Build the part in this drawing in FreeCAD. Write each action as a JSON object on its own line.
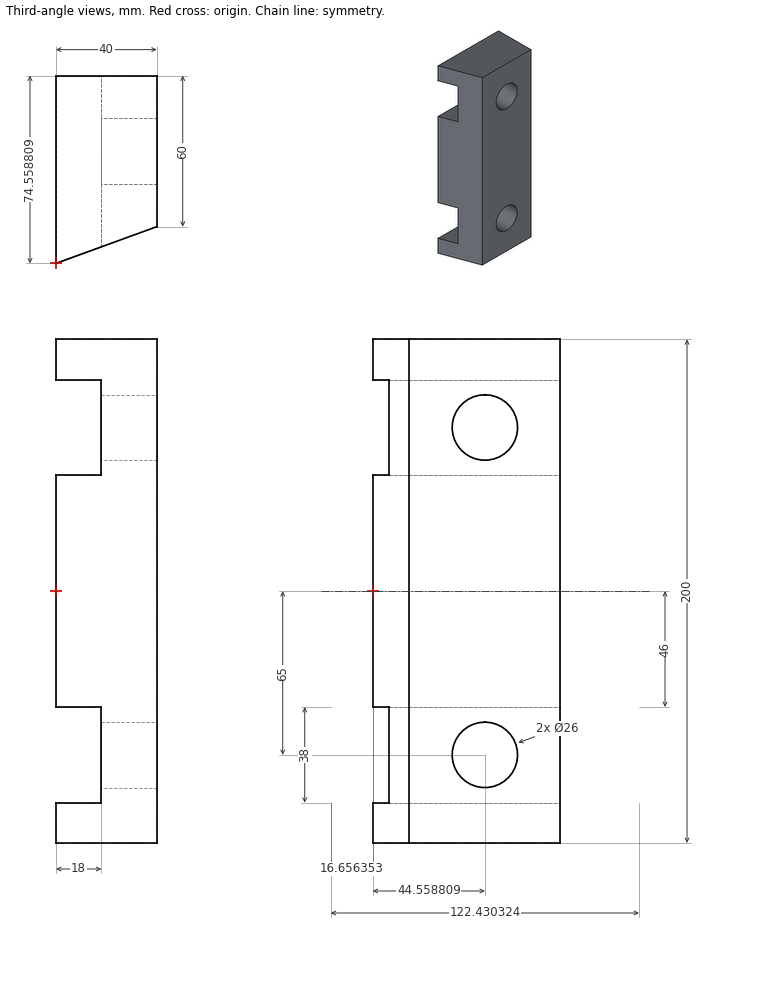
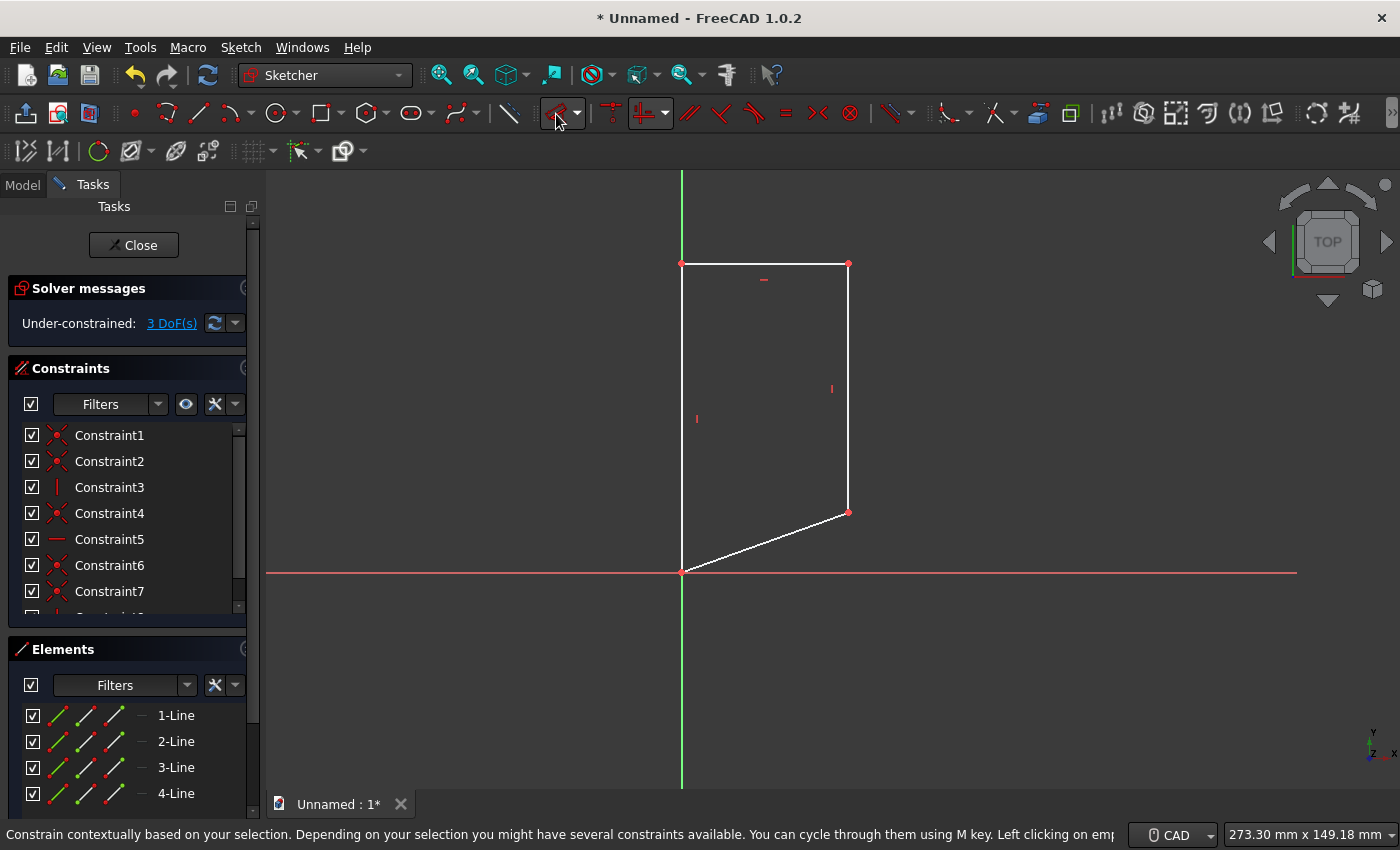
{"action": "left_click", "coordinate": [848, 438]}
{"action": "left_click", "coordinate": [882, 389]}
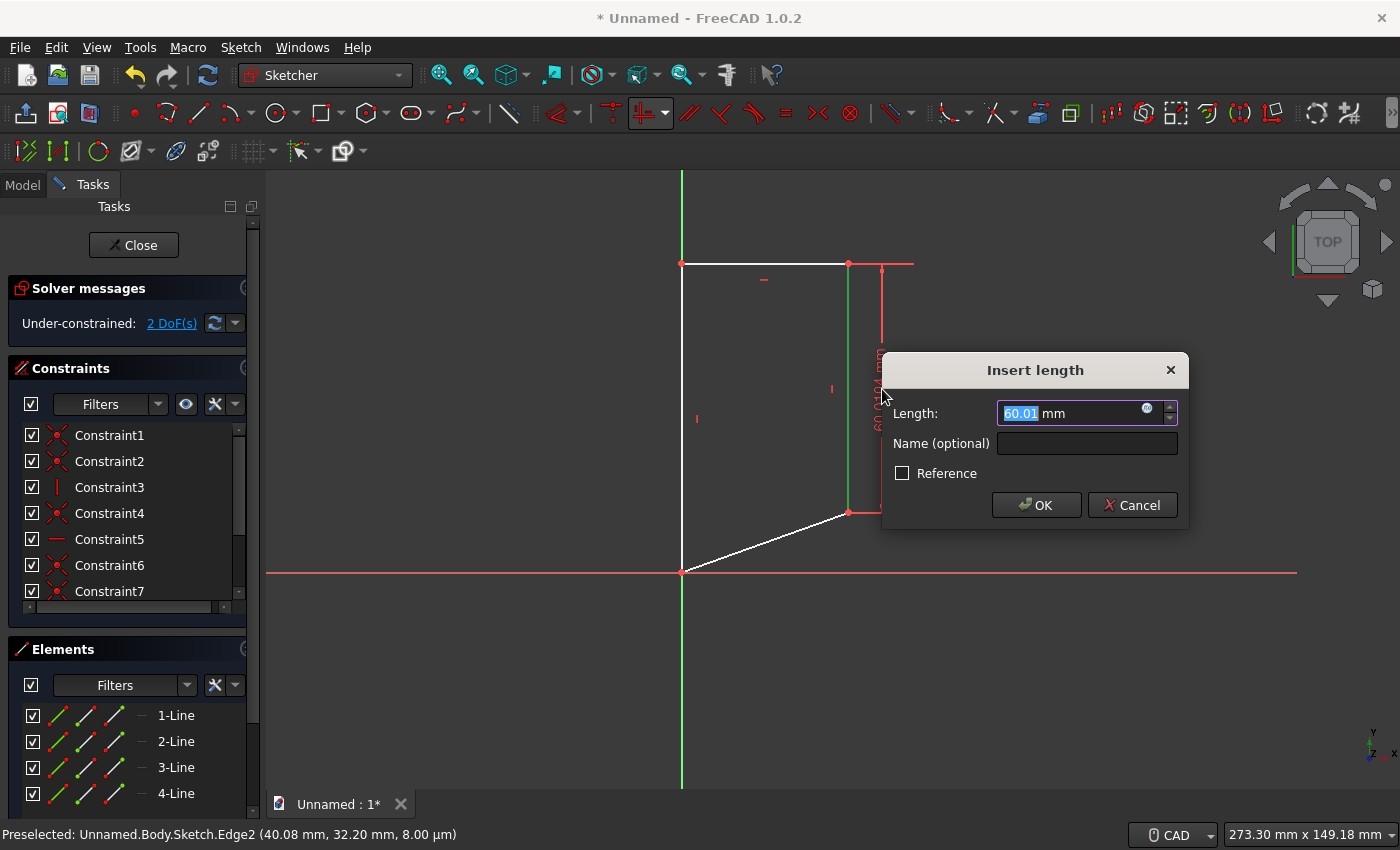
{"action": "type", "text": "60"}
{"action": "key", "text": "Return"}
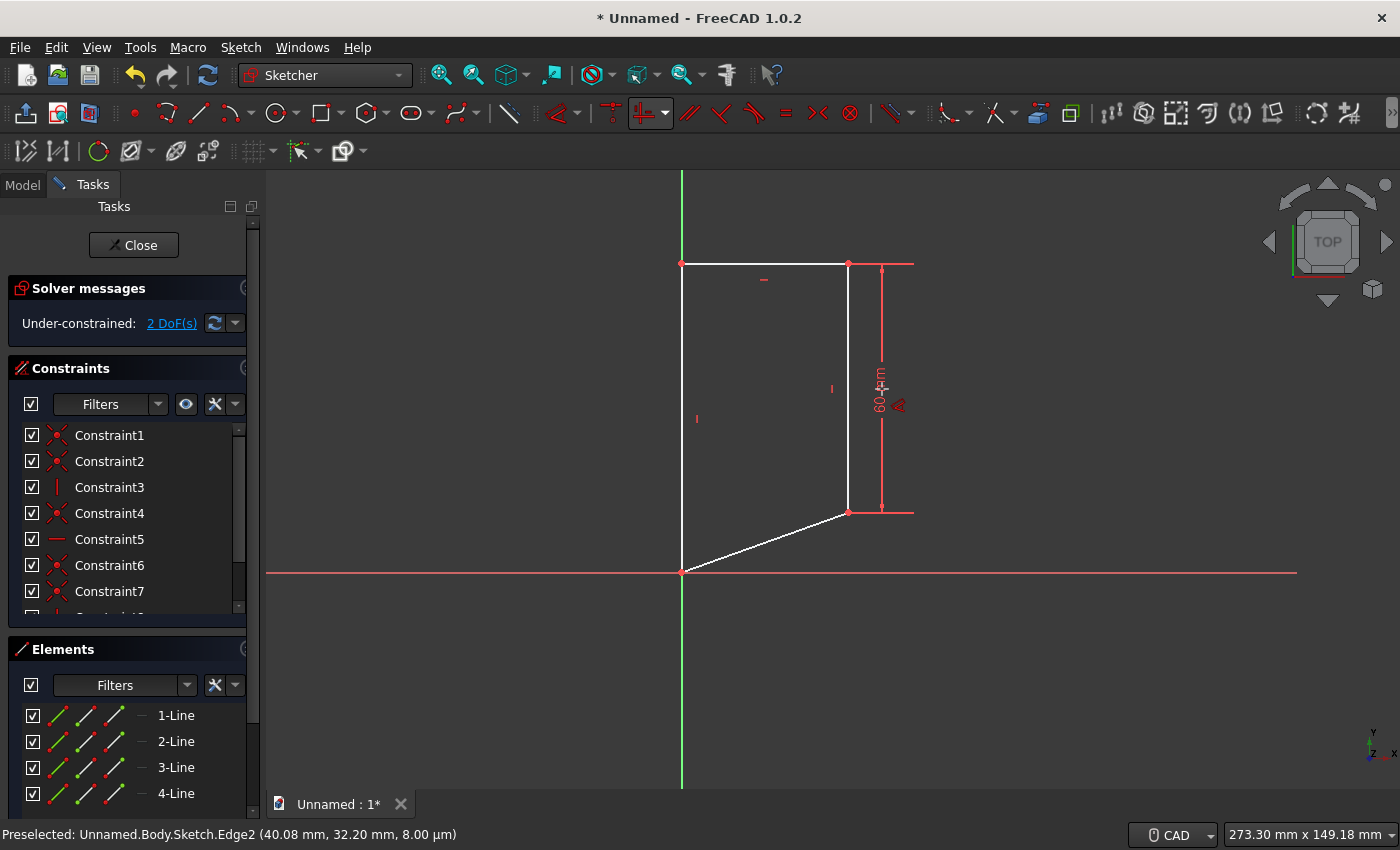
{"action": "left_click", "coordinate": [798, 264]}
{"action": "left_click", "coordinate": [765, 230]}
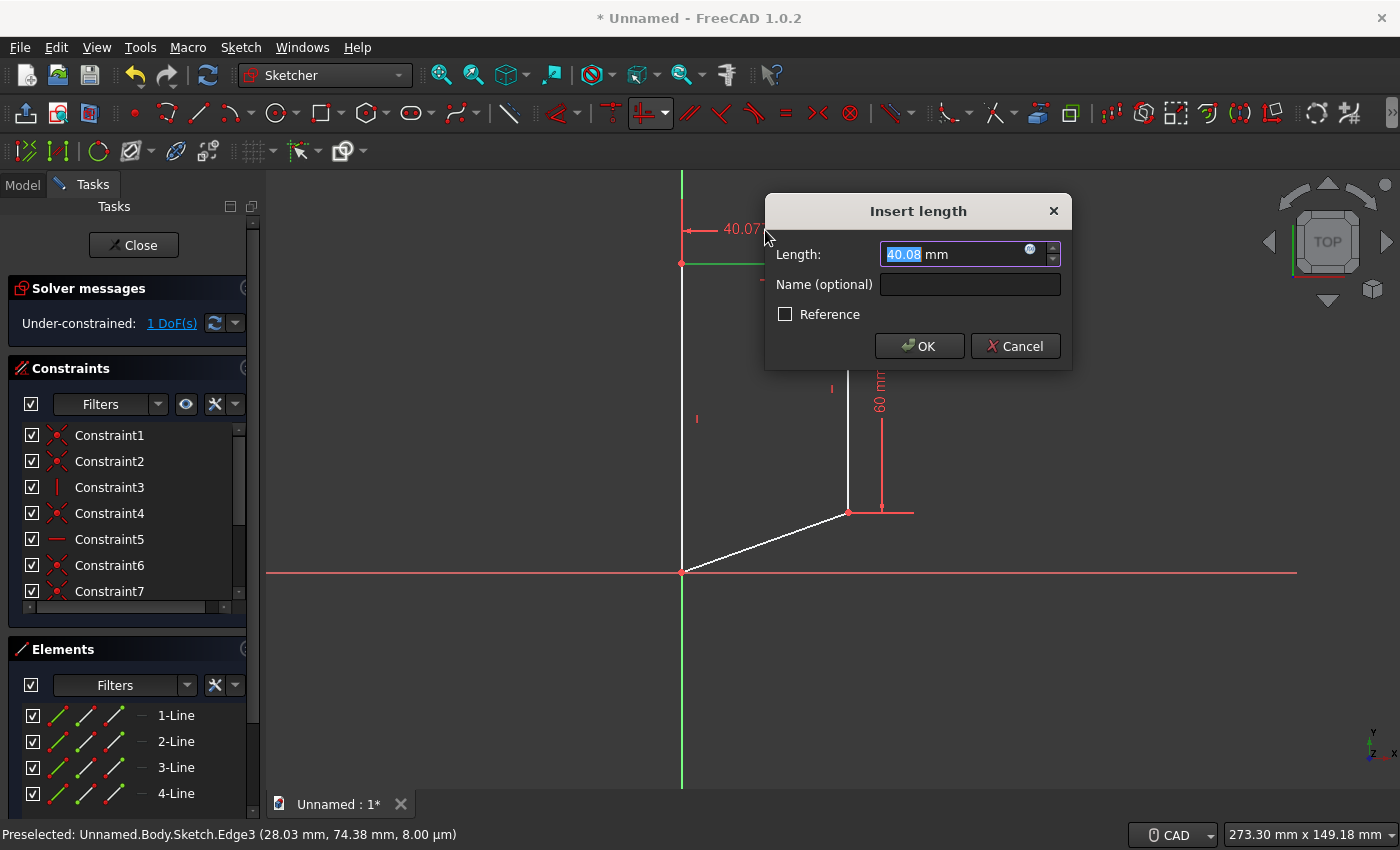
{"action": "type", "text": "40"}
{"action": "key", "text": "Return"}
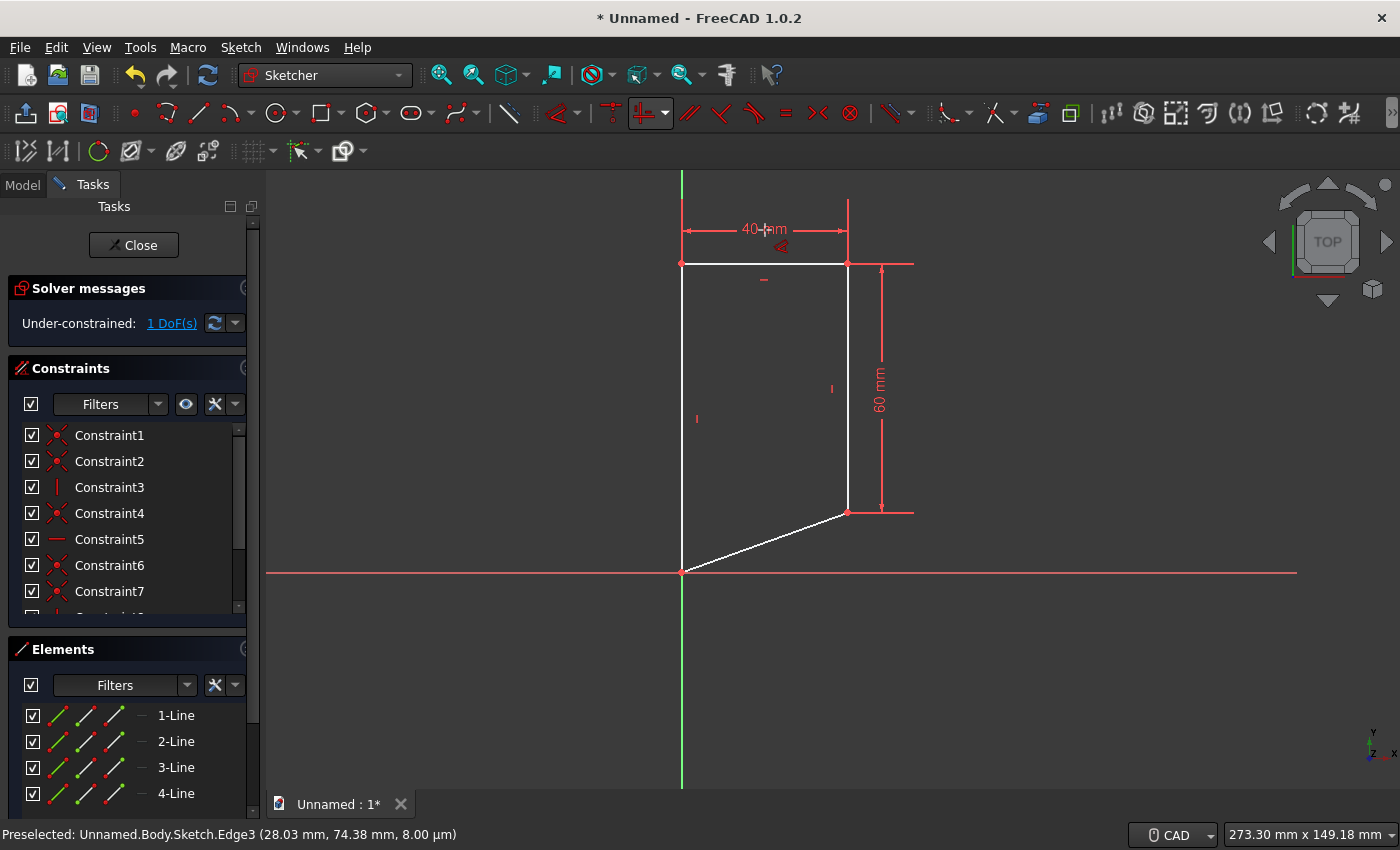
{"action": "left_click", "coordinate": [682, 357]}
{"action": "left_click", "coordinate": [648, 418]}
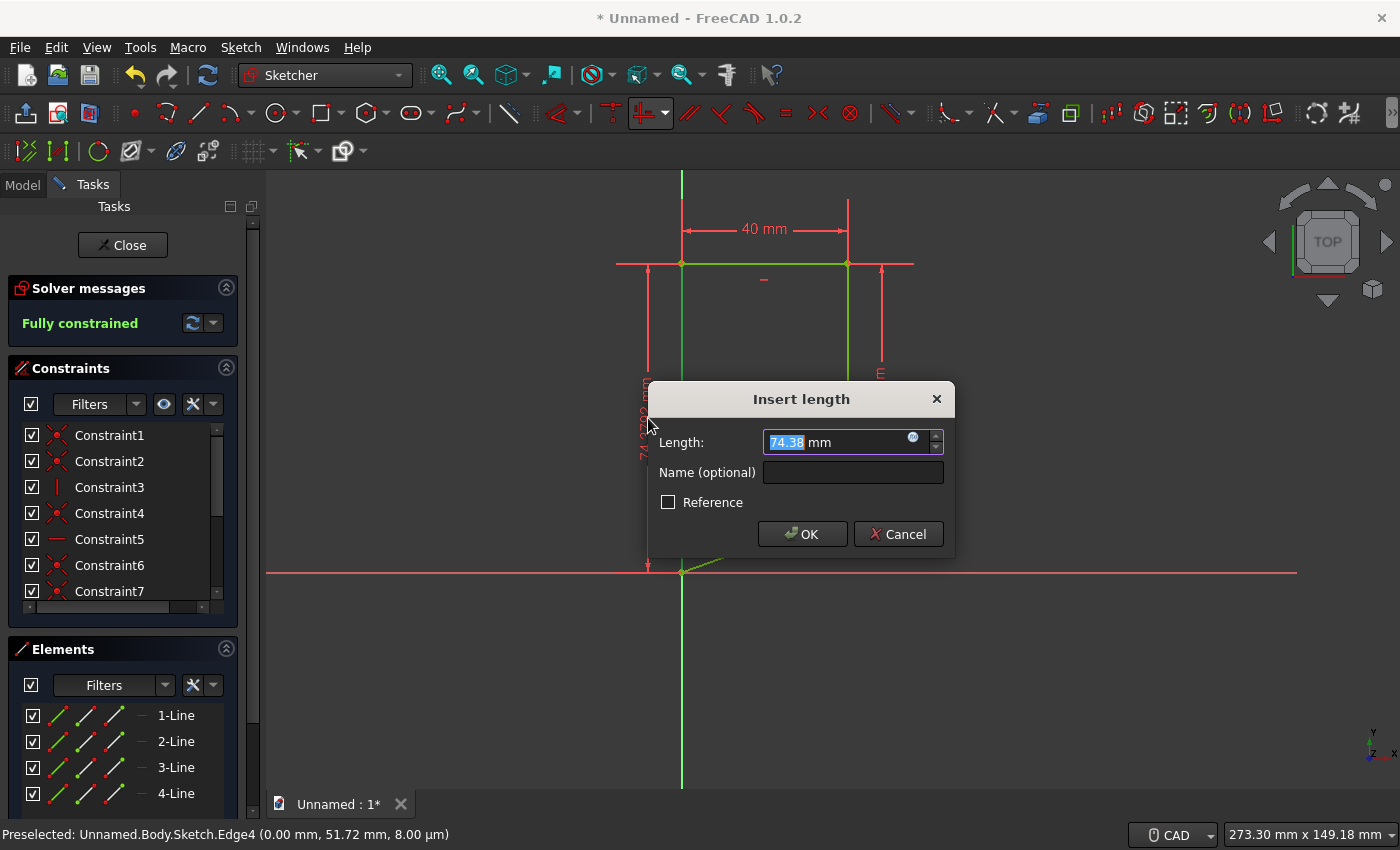
{"action": "type", "text": "74.558809"}
{"action": "key", "text": "Return"}
{"action": "key", "text": "Escape"}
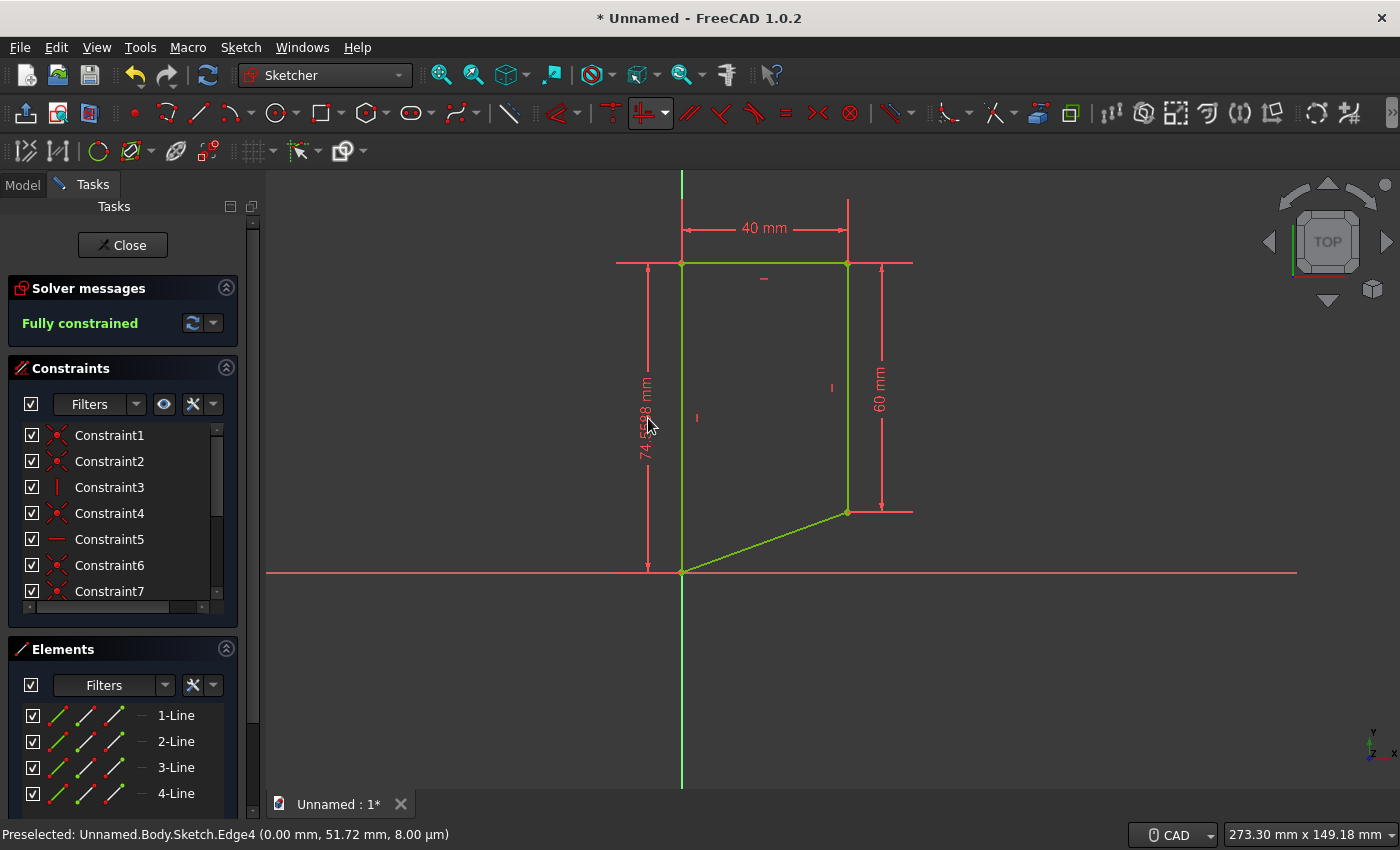
{"action": "left_click", "coordinate": [123, 245]}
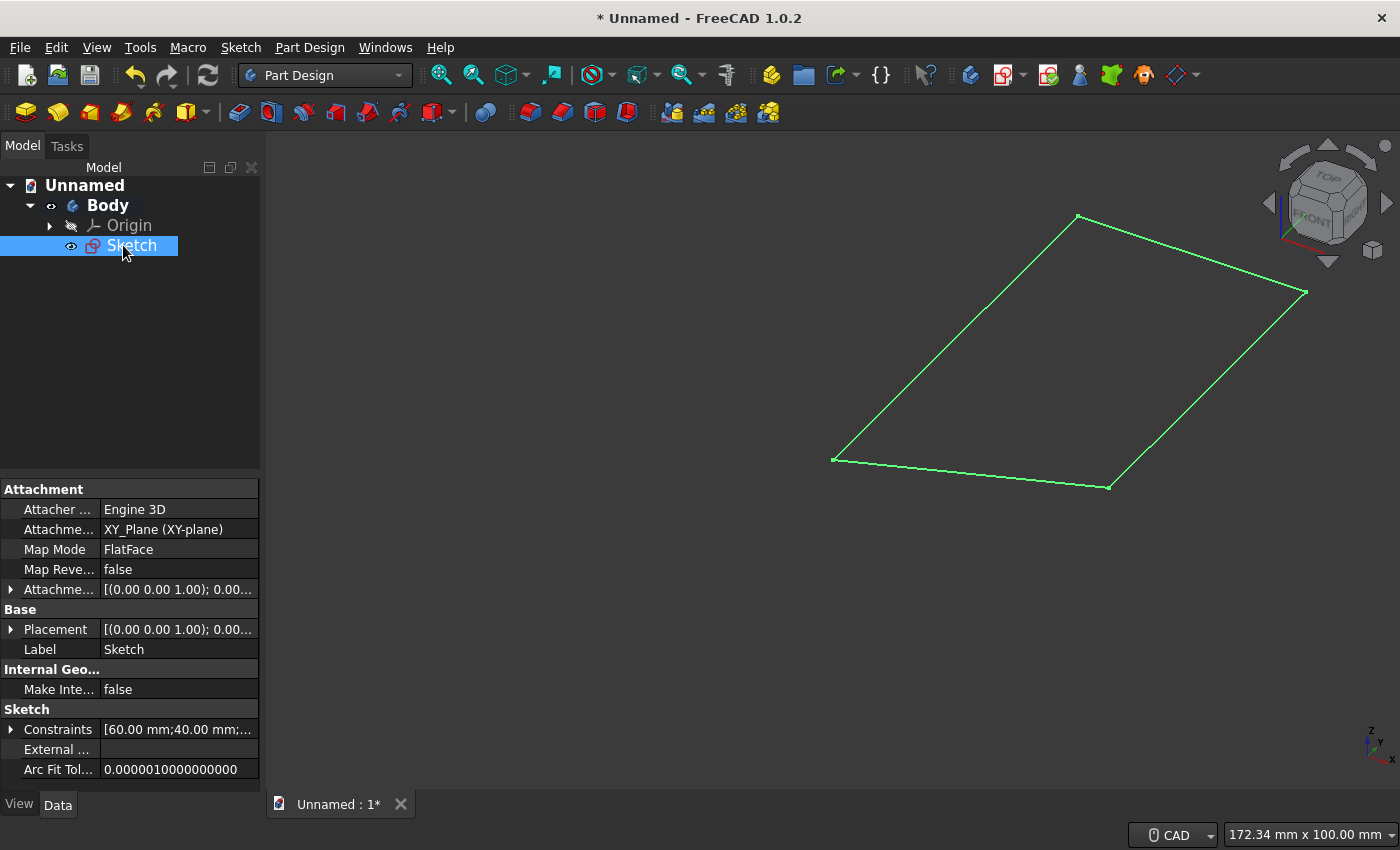
{"action": "left_click", "coordinate": [26, 112]}